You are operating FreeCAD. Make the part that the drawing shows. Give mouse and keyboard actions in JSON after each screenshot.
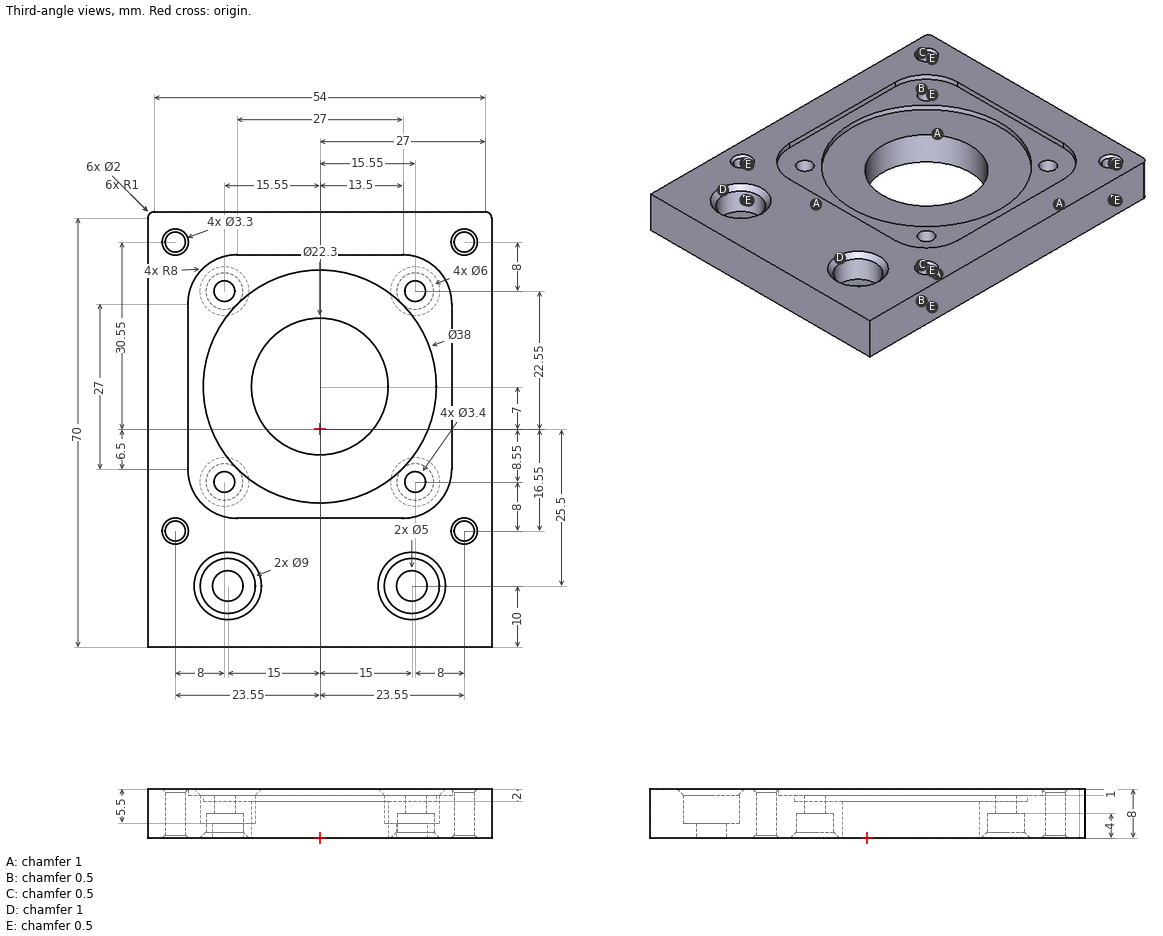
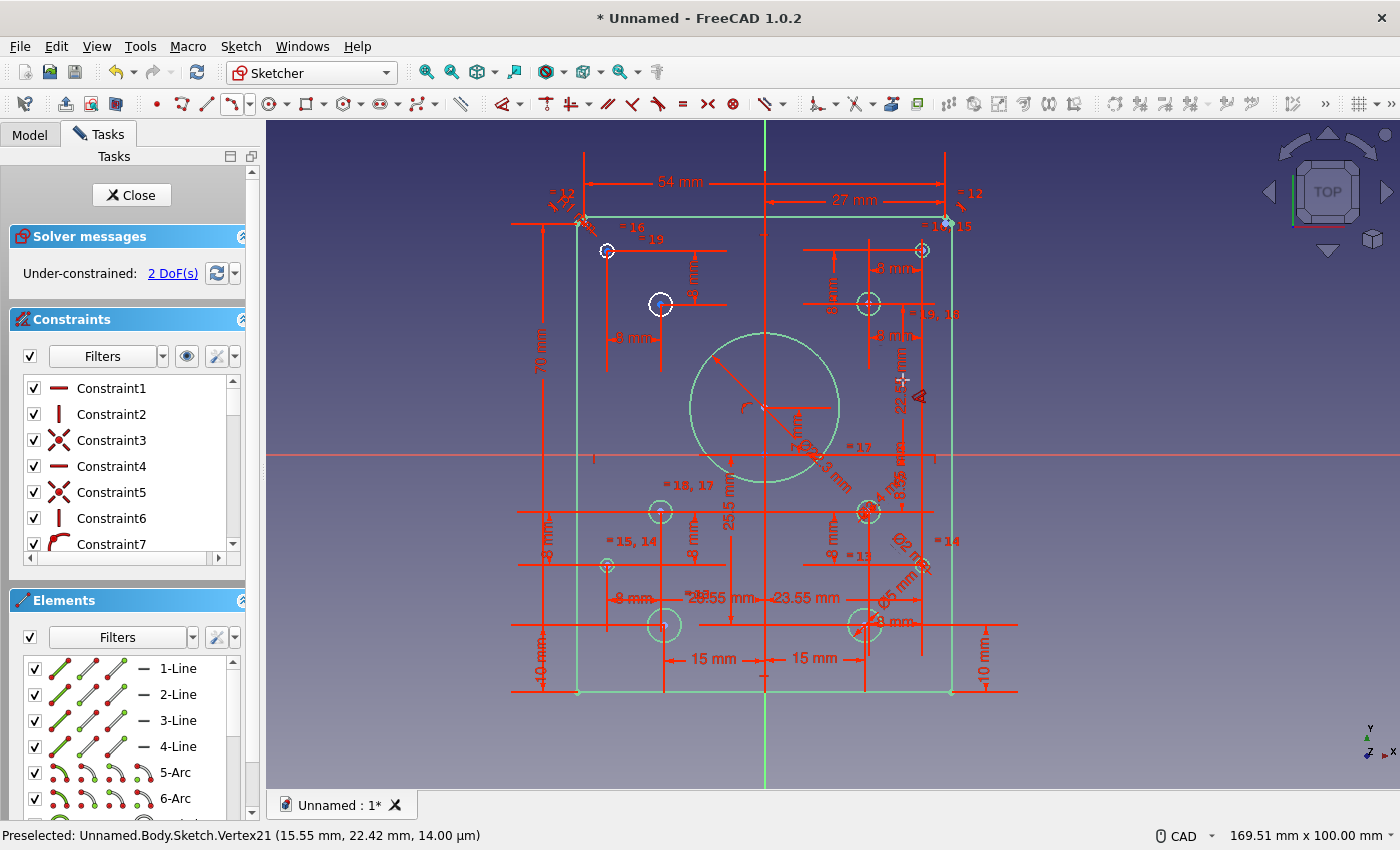
{"action": "left_click", "coordinate": [661, 305]}
{"action": "left_click", "coordinate": [713, 247]}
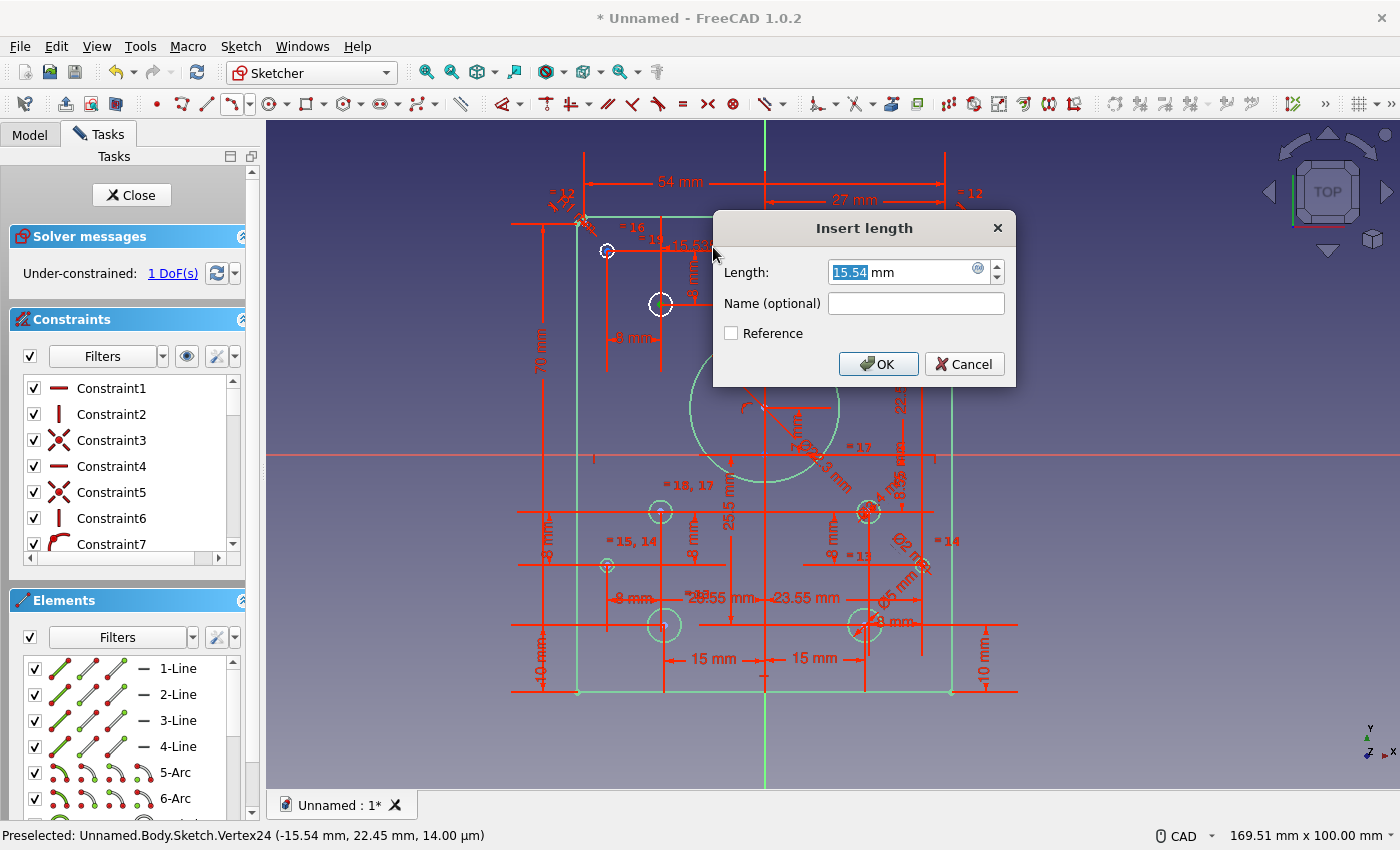
{"action": "type", "text": "15.55"}
{"action": "key", "text": "Return"}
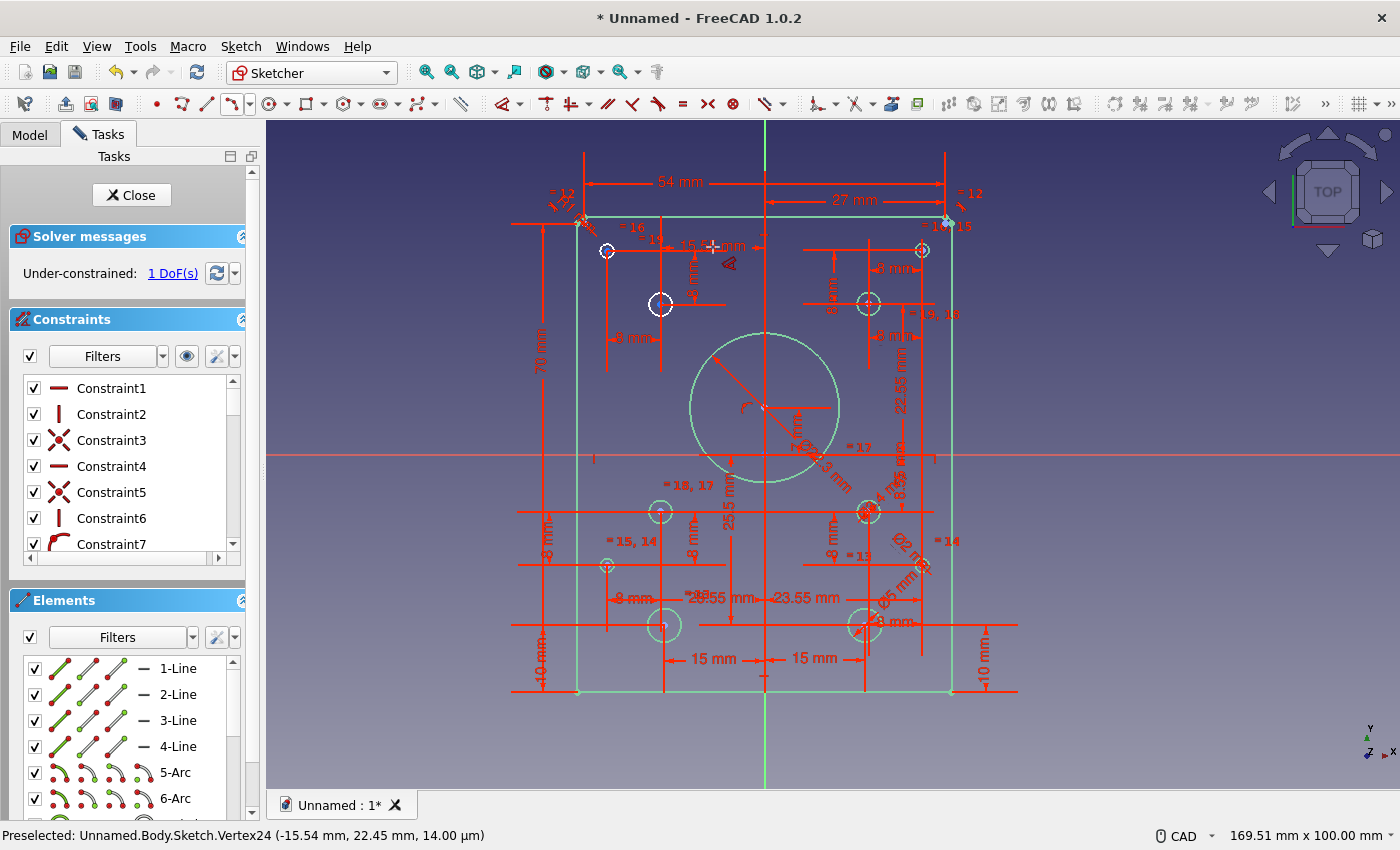
{"action": "left_click", "coordinate": [661, 305]}
{"action": "left_click", "coordinate": [627, 380]}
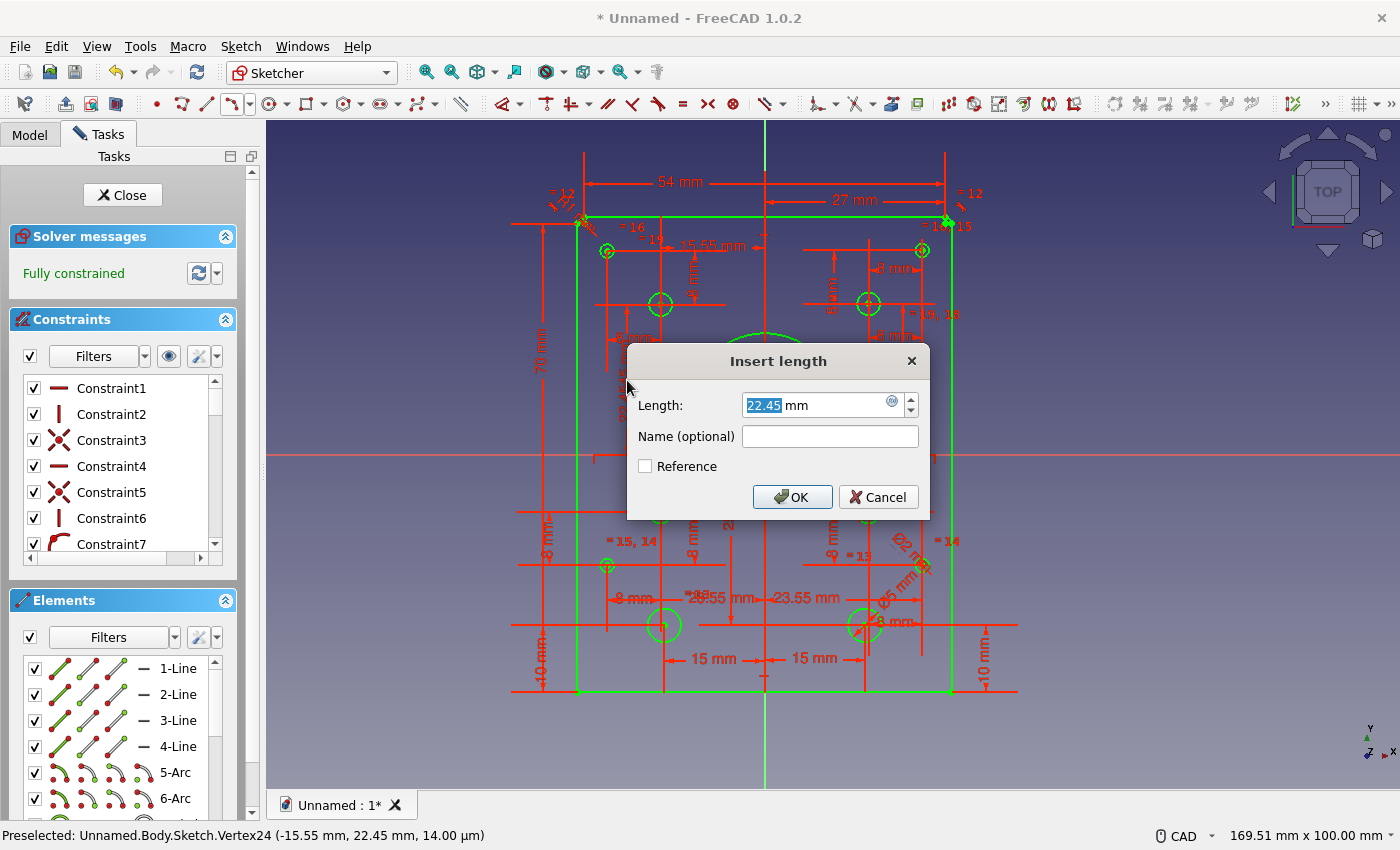
{"action": "type", "text": "22.55"}
{"action": "key", "text": "Return"}
{"action": "key", "text": "Escape"}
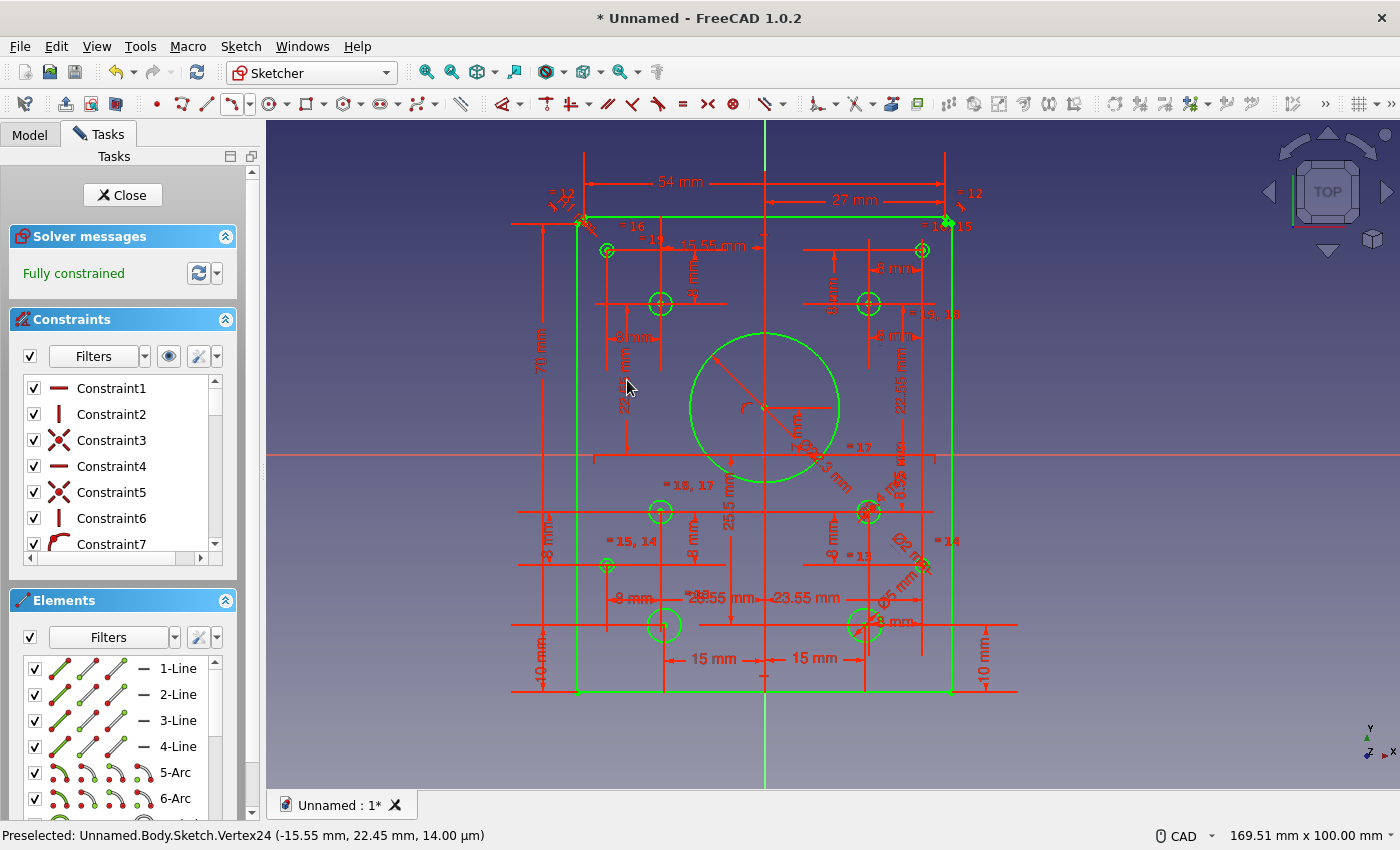
{"action": "left_click", "coordinate": [123, 195]}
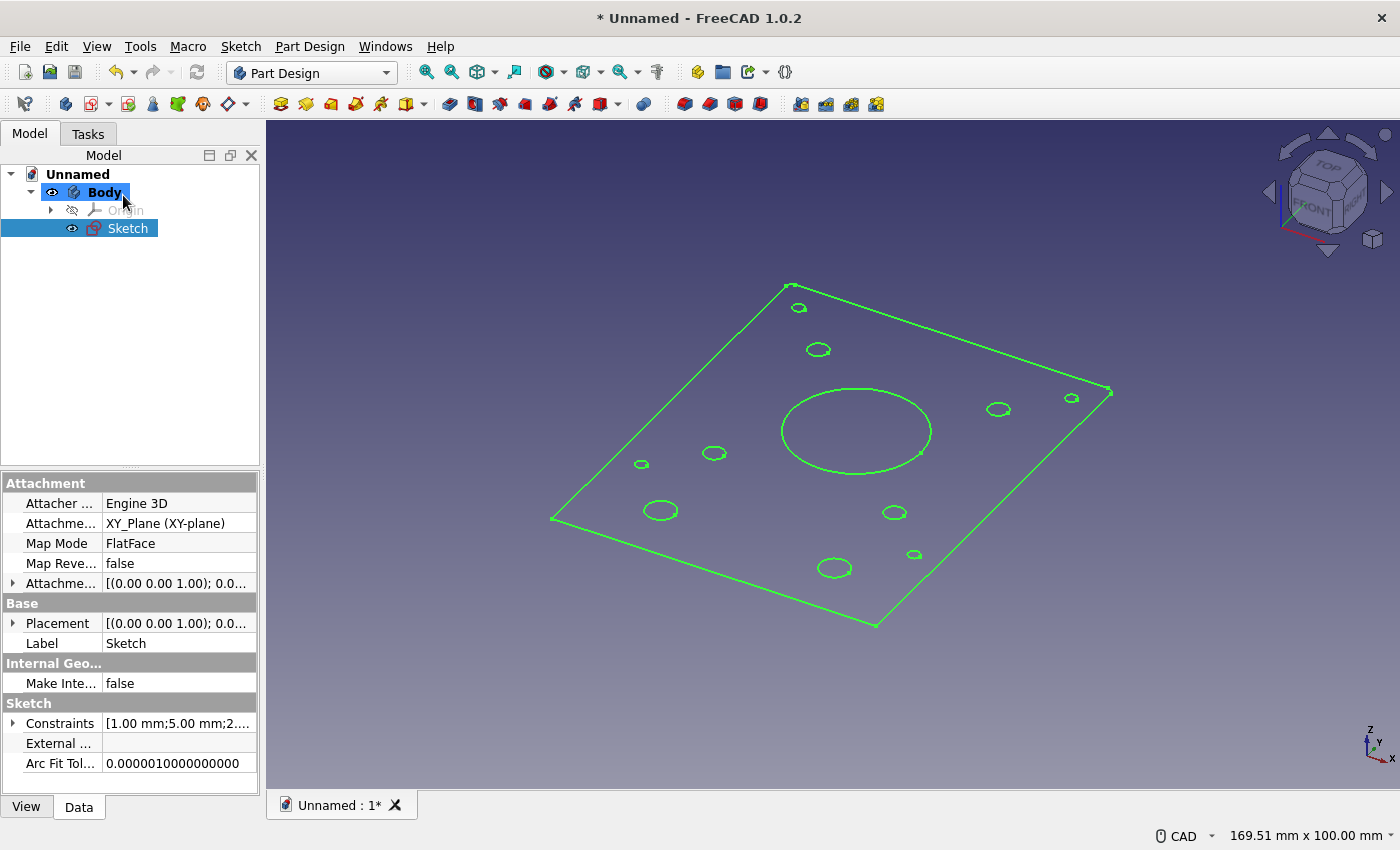
{"action": "left_click", "coordinate": [281, 104]}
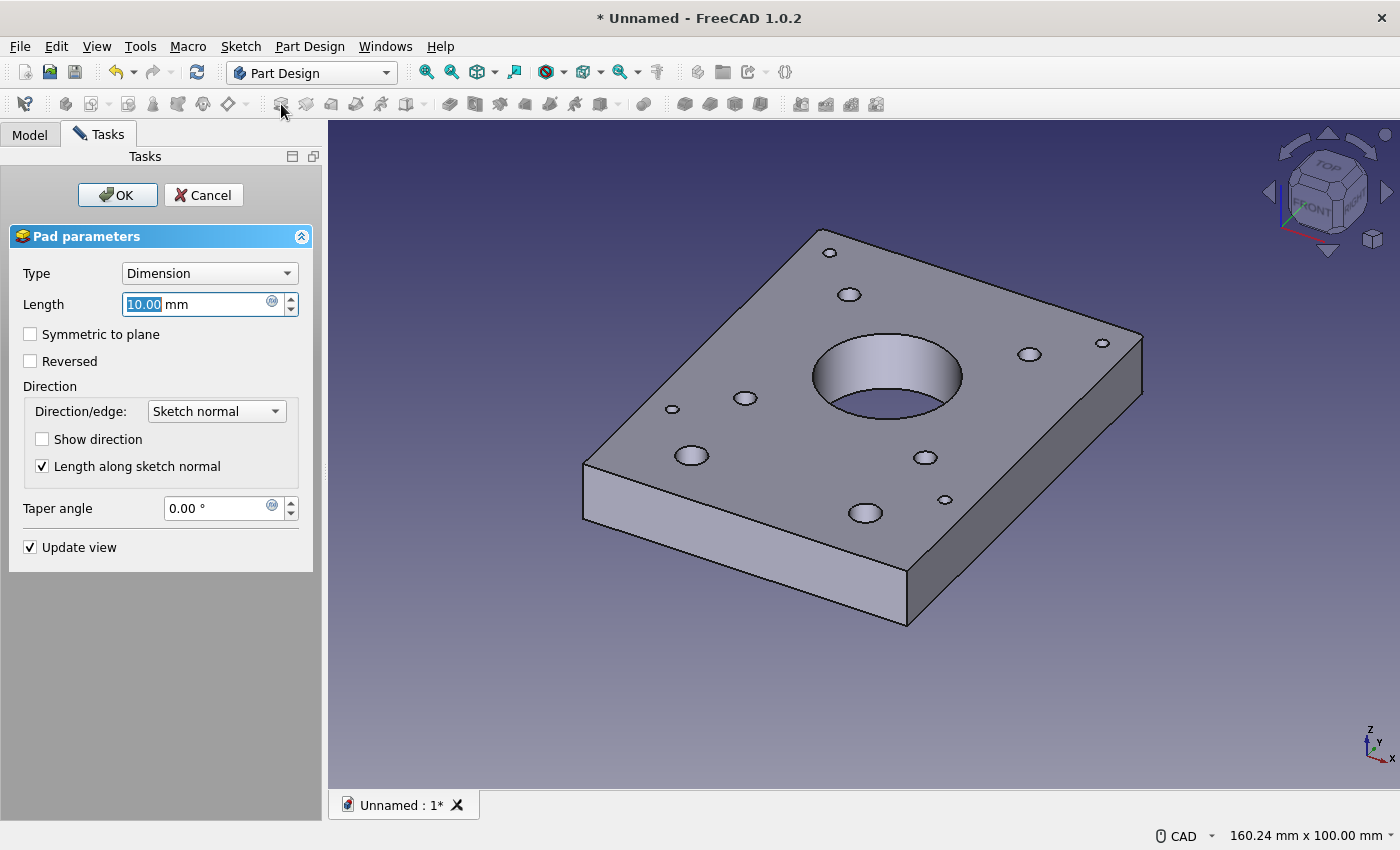
{"action": "type", "text": "8"}
{"action": "key", "text": "Tab"}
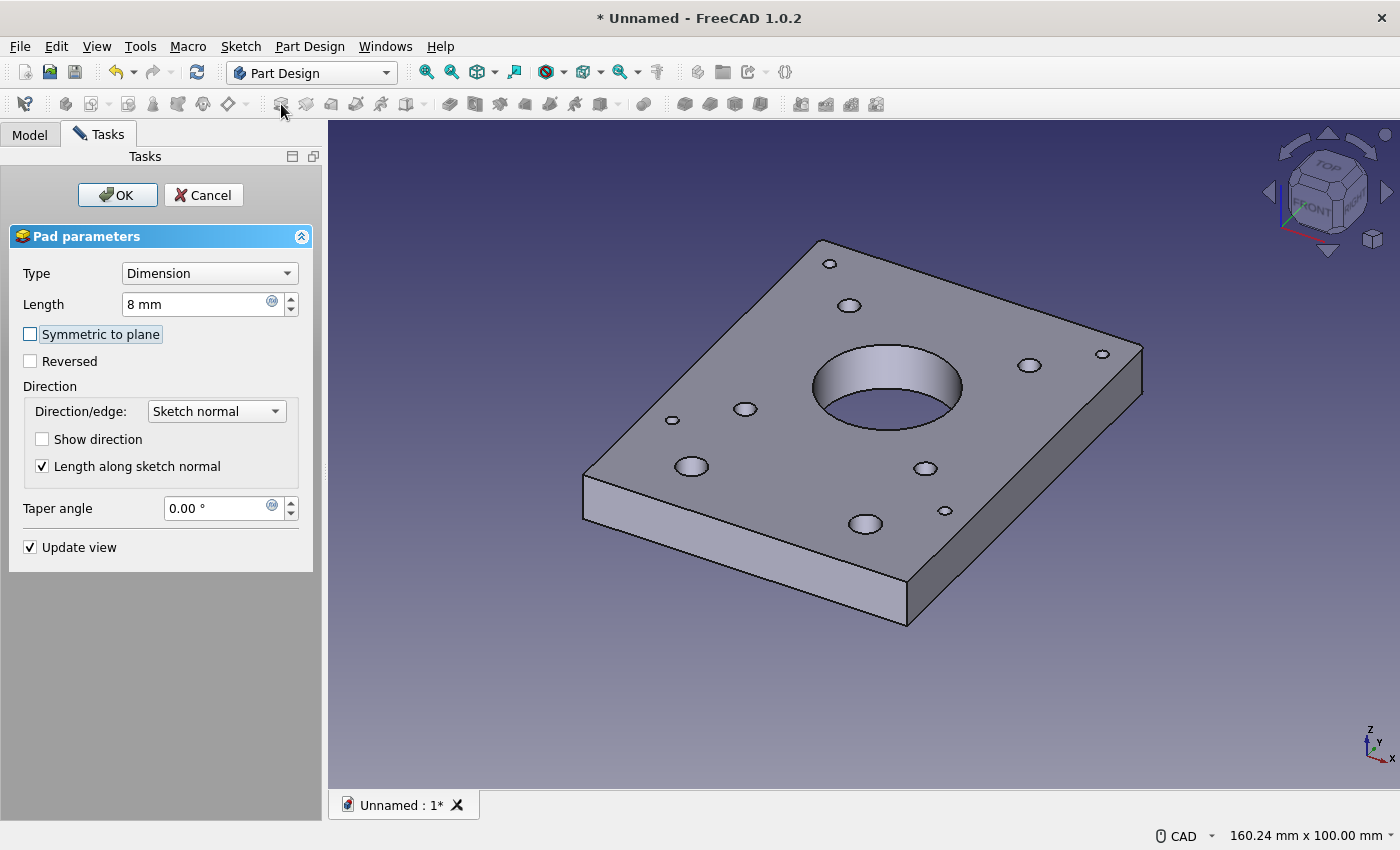
{"action": "left_click", "coordinate": [118, 195]}